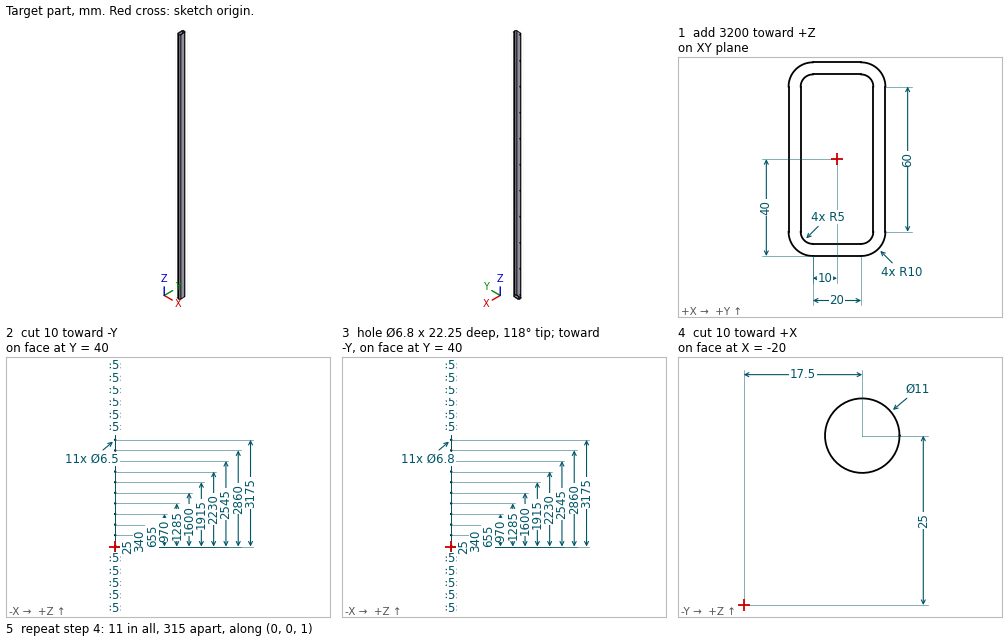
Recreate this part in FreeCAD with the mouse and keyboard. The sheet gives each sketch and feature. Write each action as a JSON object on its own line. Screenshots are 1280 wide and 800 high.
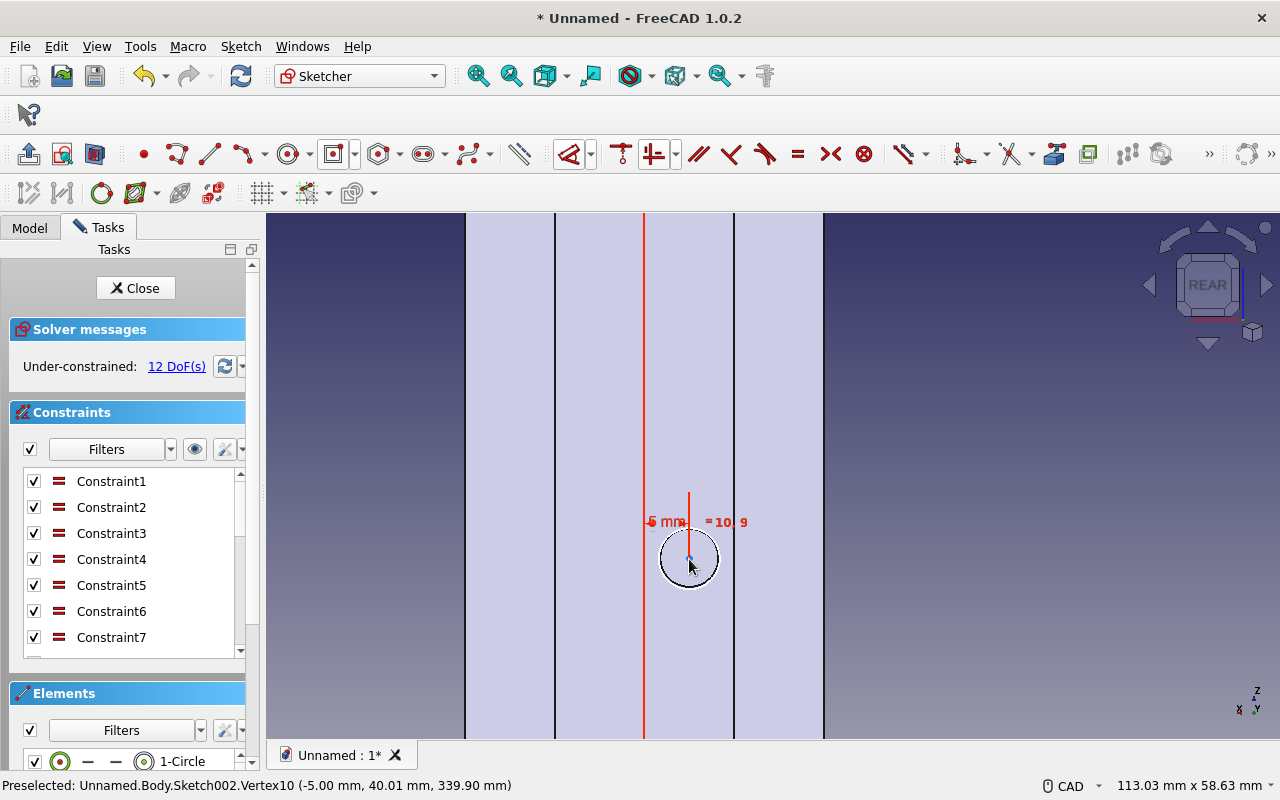
{"action": "scroll", "coordinate": [704, 476], "scroll_direction": "down", "scroll_amount": 15}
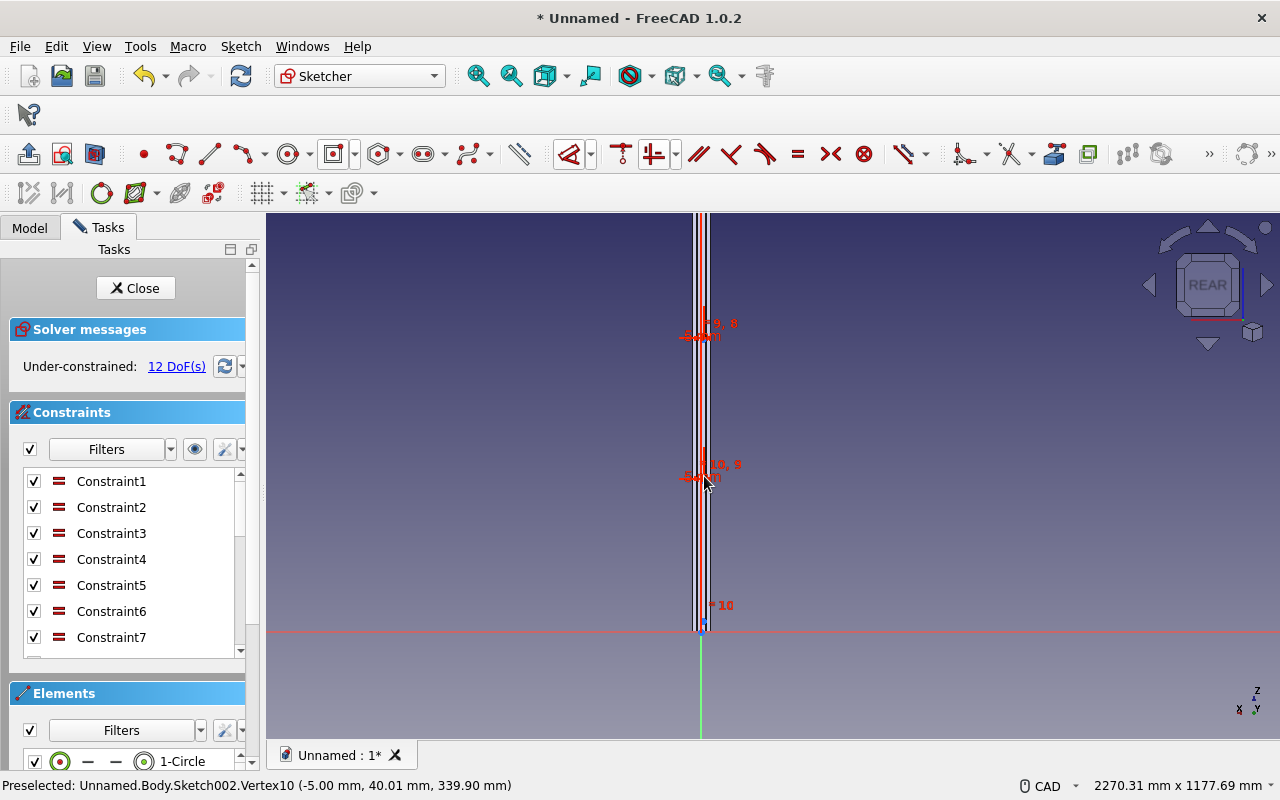
{"action": "scroll", "coordinate": [705, 657], "scroll_direction": "down", "scroll_amount": 7}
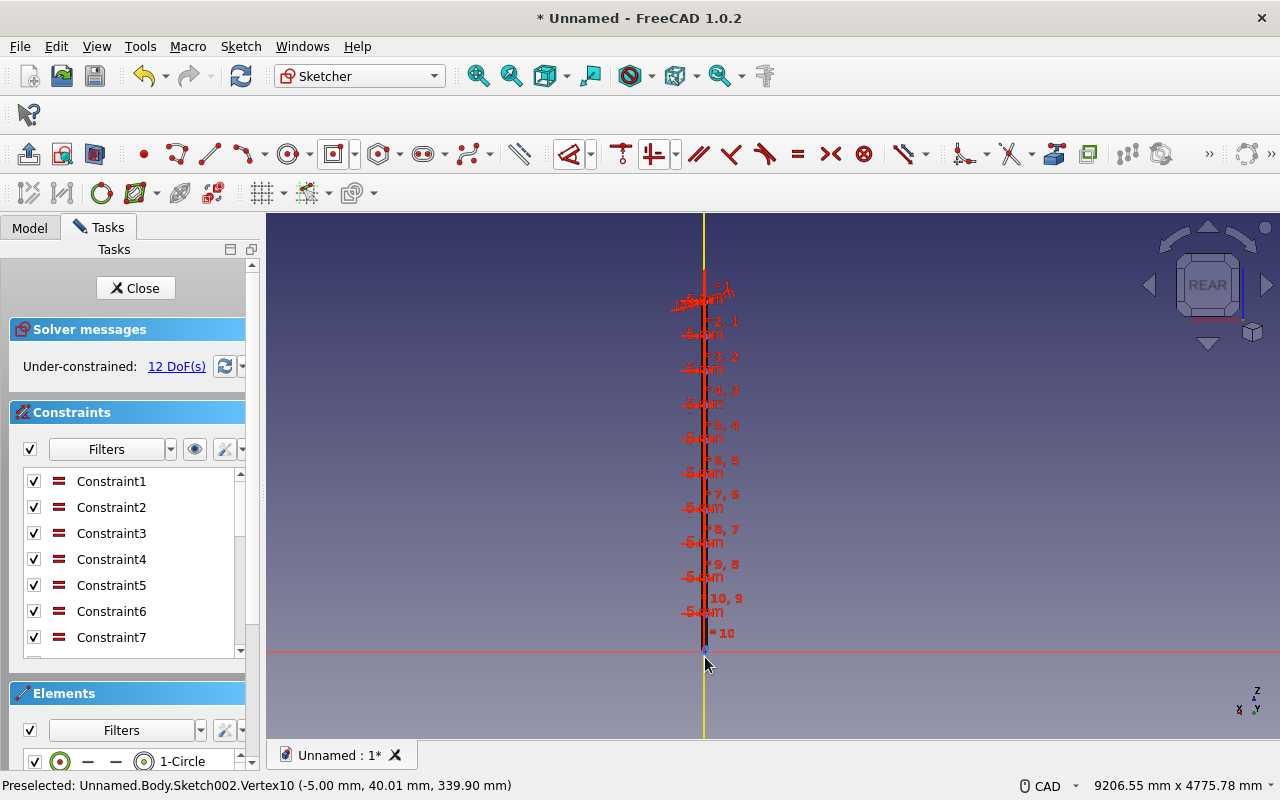
{"action": "scroll", "coordinate": [705, 649], "scroll_direction": "up", "scroll_amount": 22}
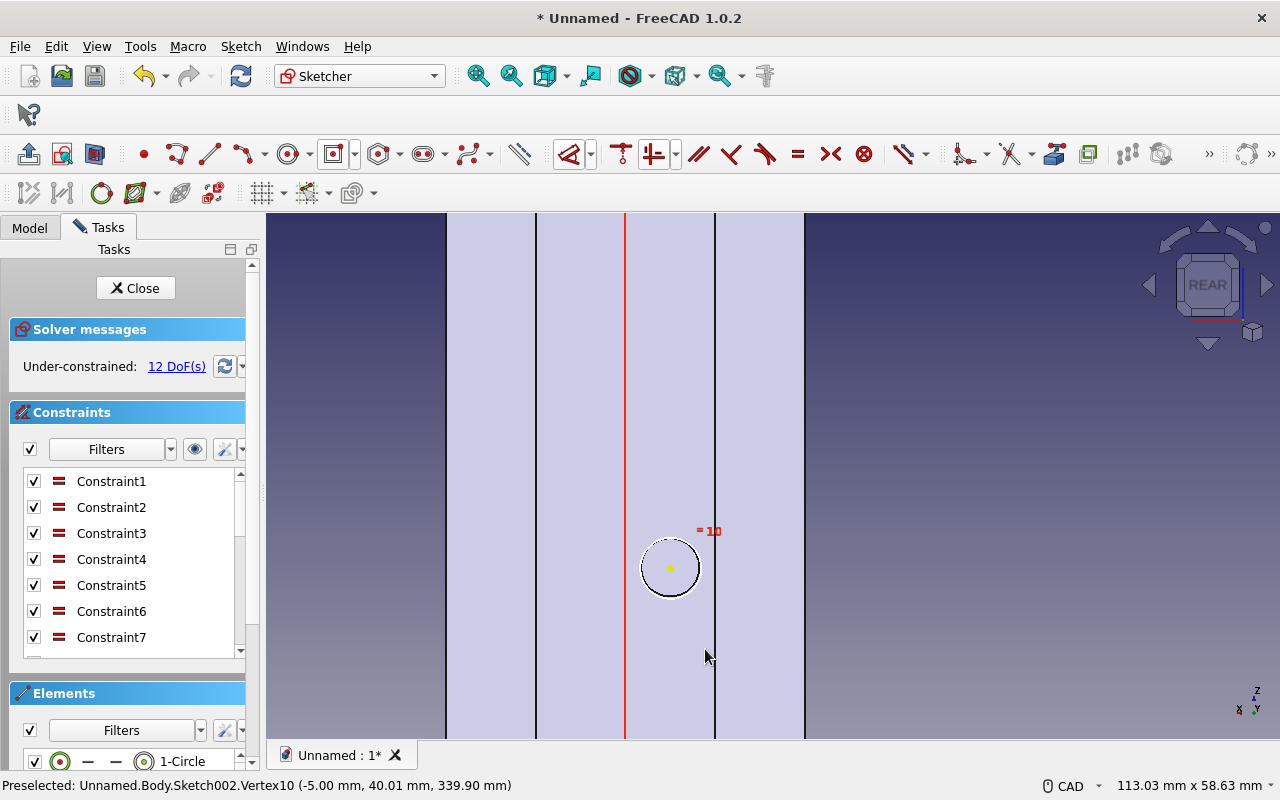
{"action": "left_click", "coordinate": [671, 568]}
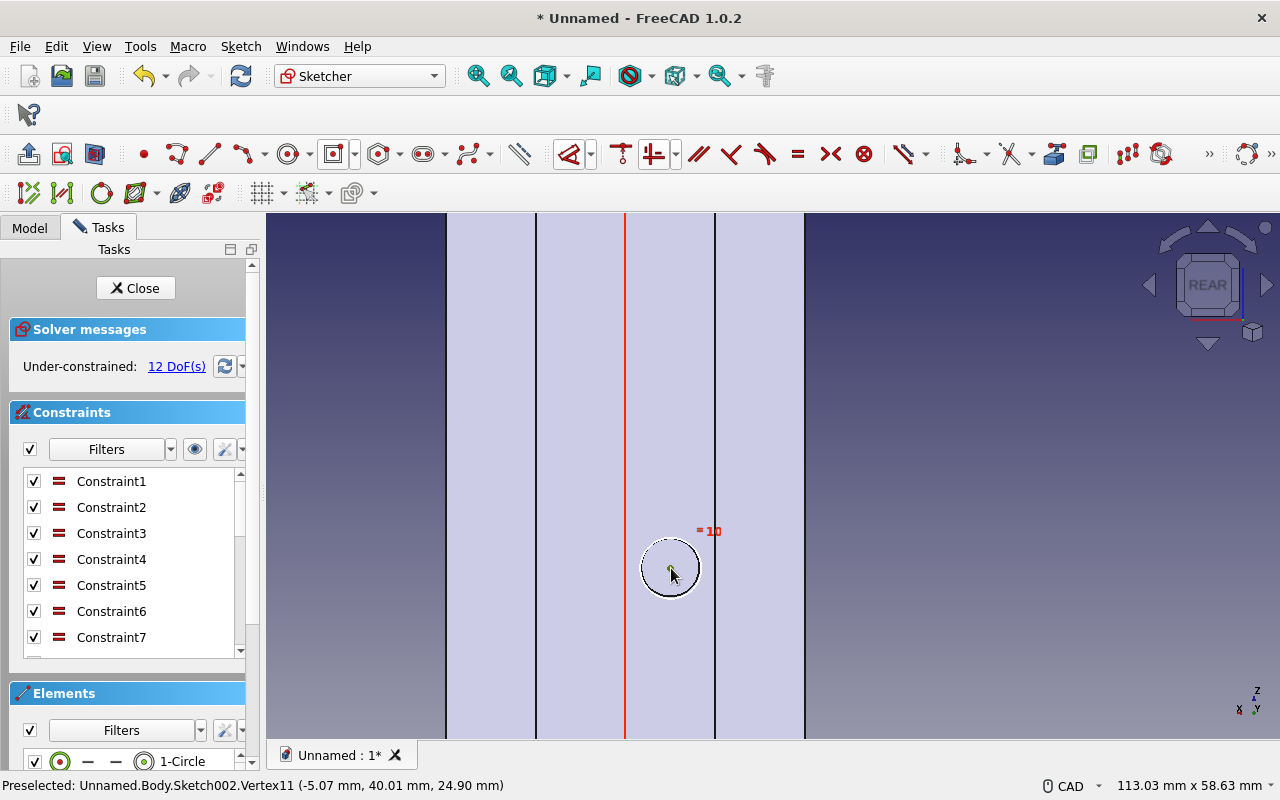
{"action": "key", "text": "l"}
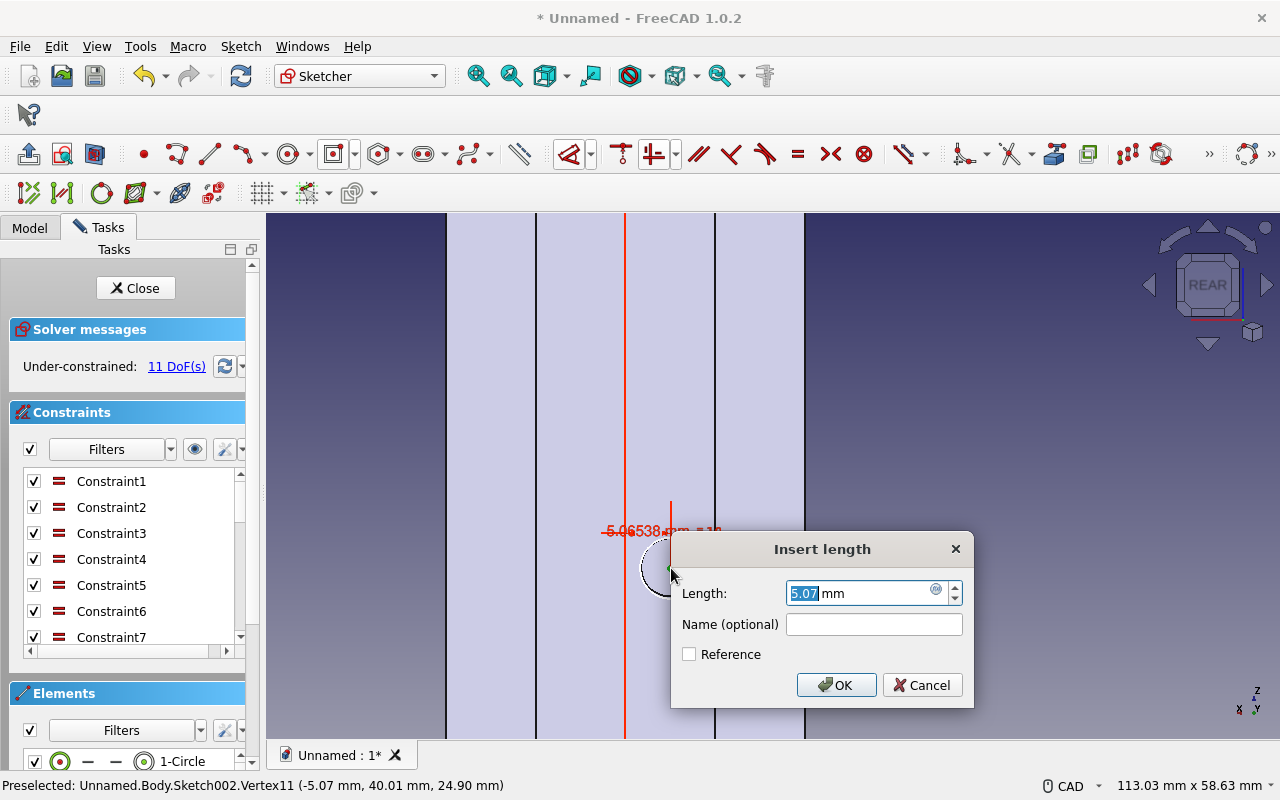
{"action": "type", "text": "5"}
{"action": "key", "text": "Return"}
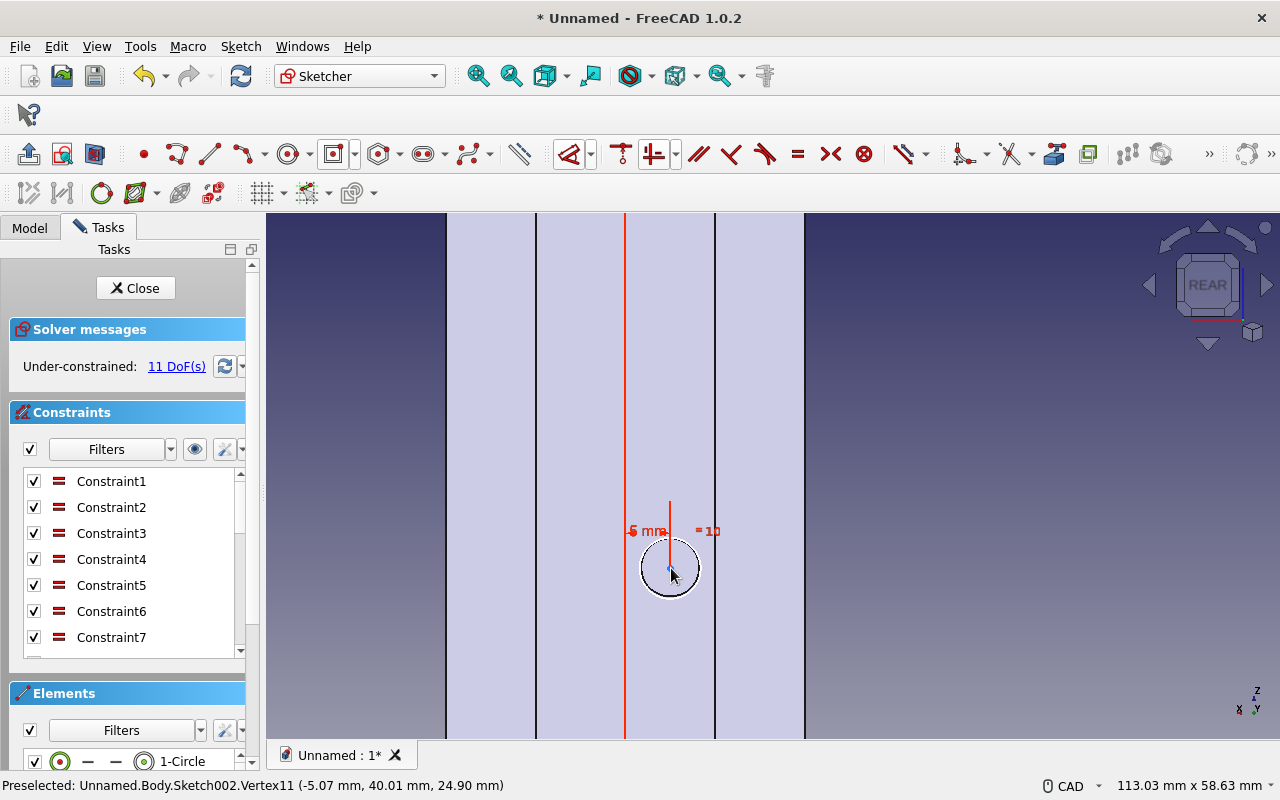
{"action": "scroll", "coordinate": [704, 476], "scroll_direction": "down", "scroll_amount": 15}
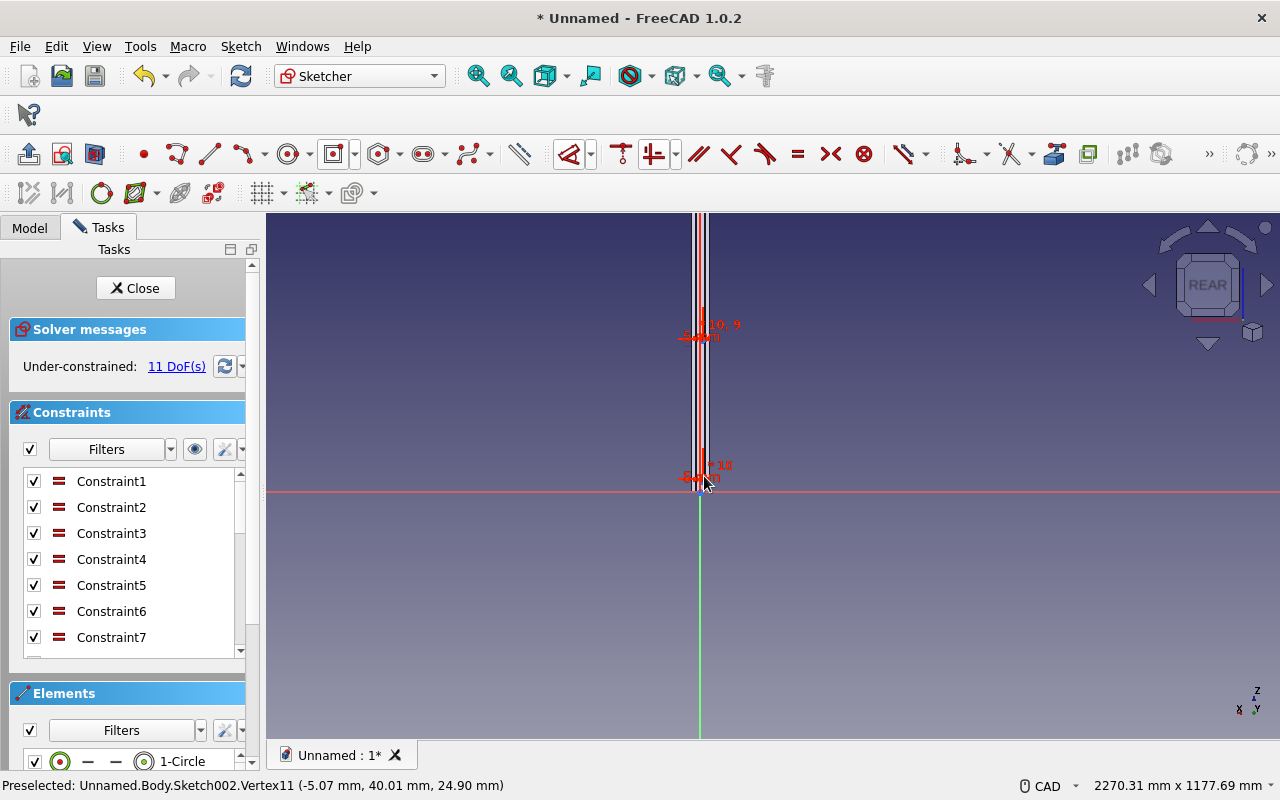
{"action": "scroll", "coordinate": [705, 703], "scroll_direction": "down", "scroll_amount": 7}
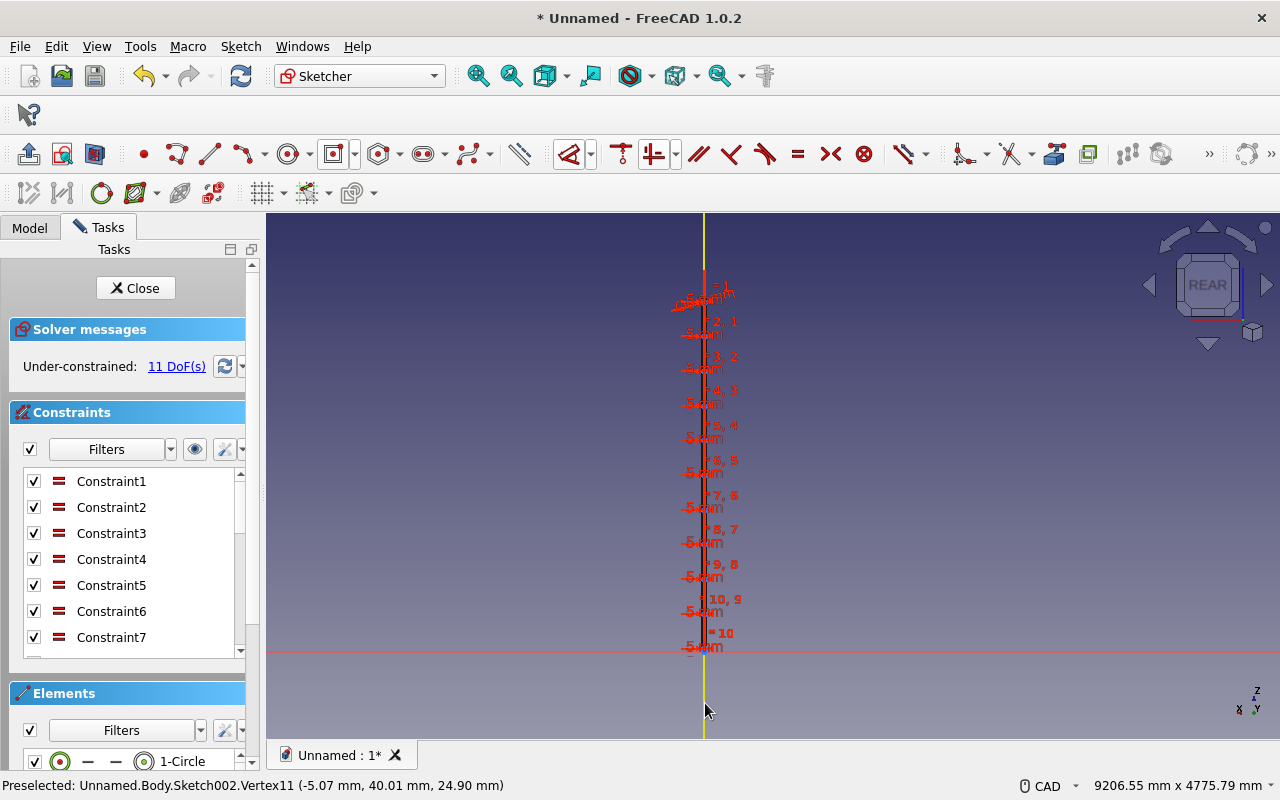
{"action": "scroll", "coordinate": [705, 649], "scroll_direction": "up", "scroll_amount": 14}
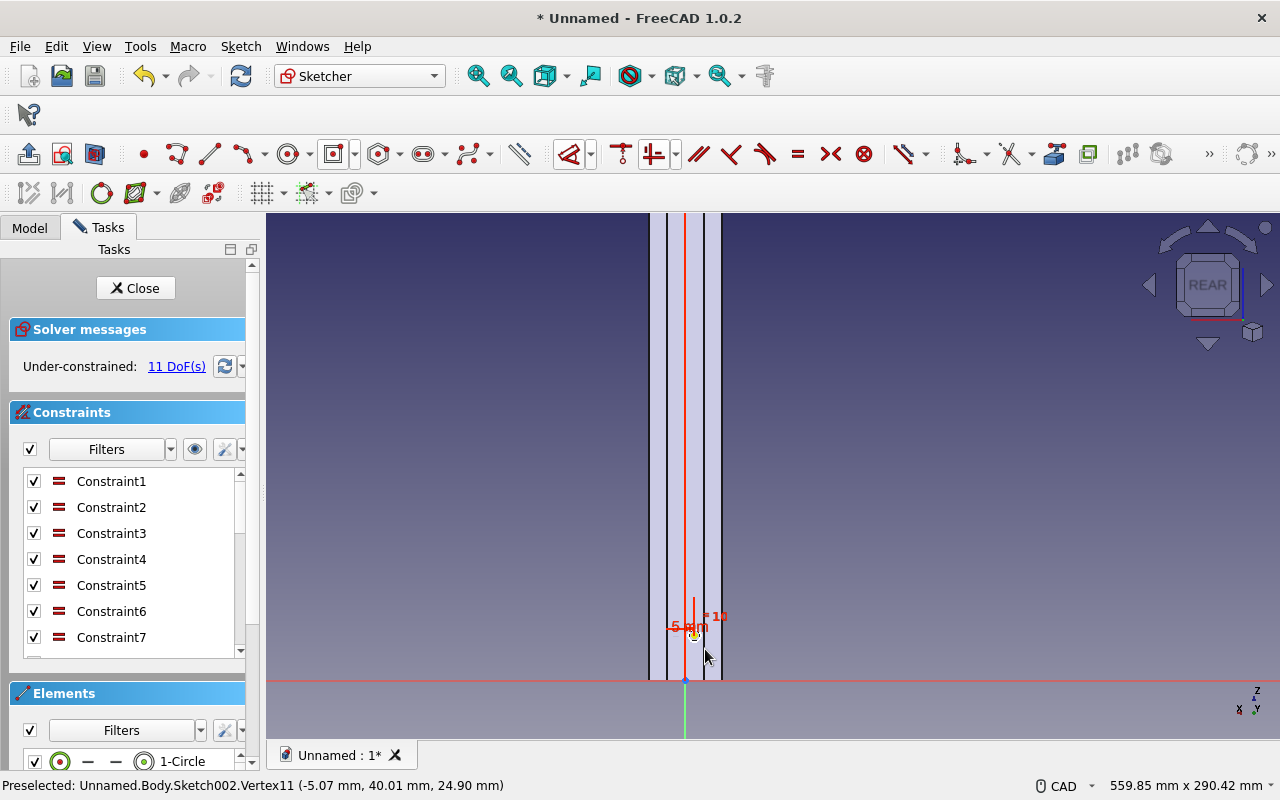
{"action": "left_click", "coordinate": [694, 636]}